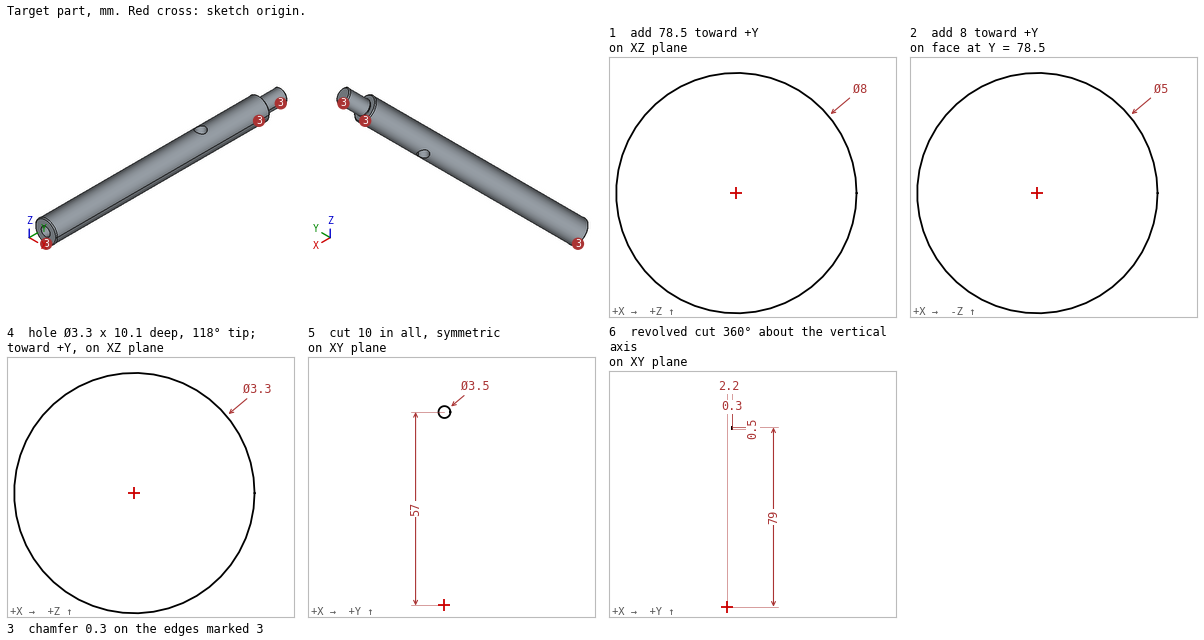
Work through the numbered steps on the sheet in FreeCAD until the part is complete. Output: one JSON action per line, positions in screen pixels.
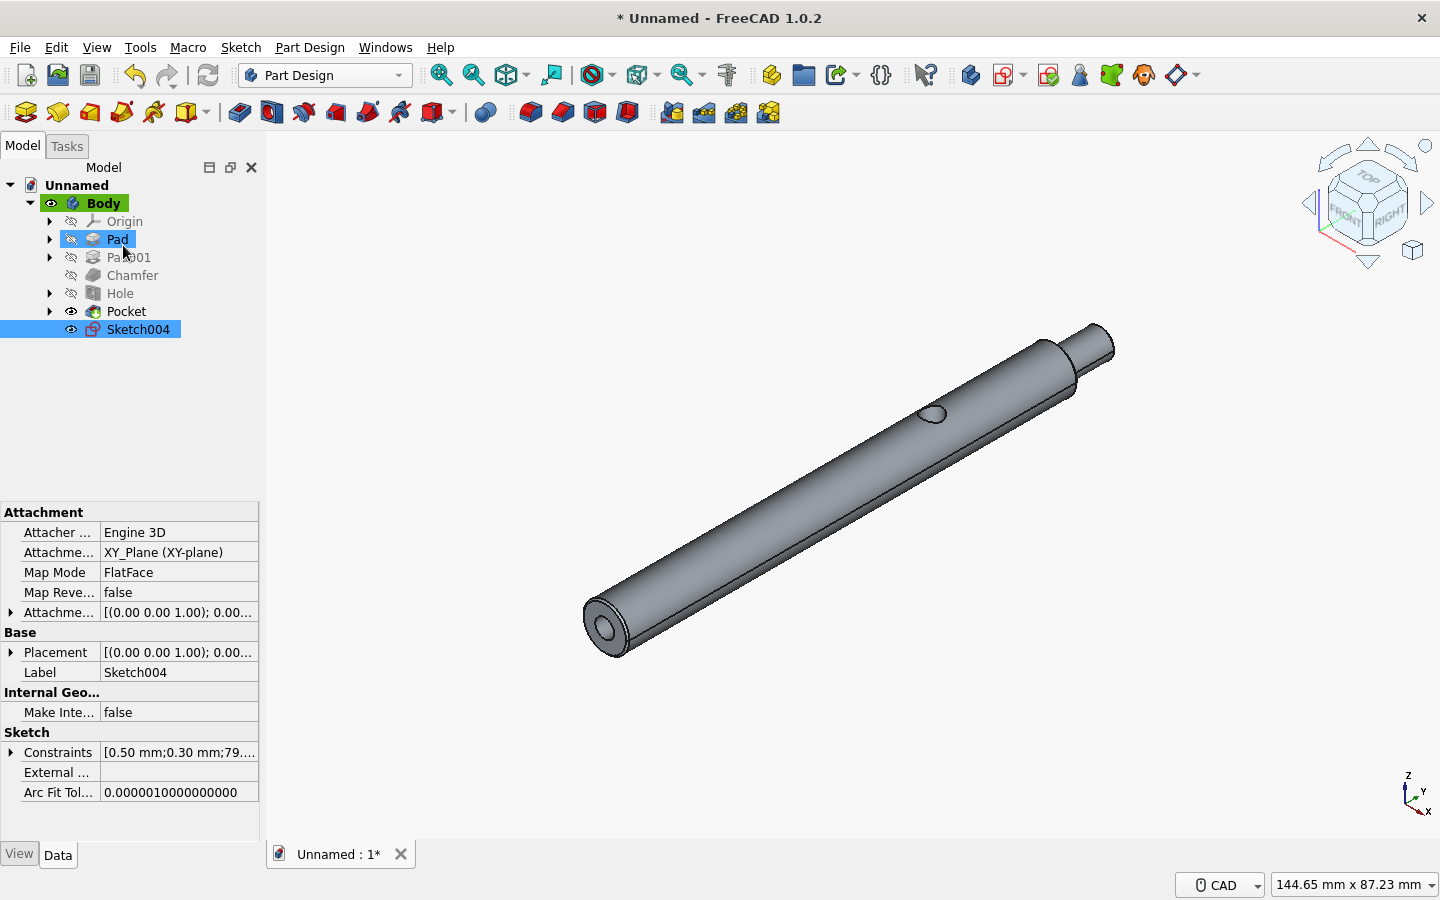
{"action": "left_click", "coordinate": [304, 112]}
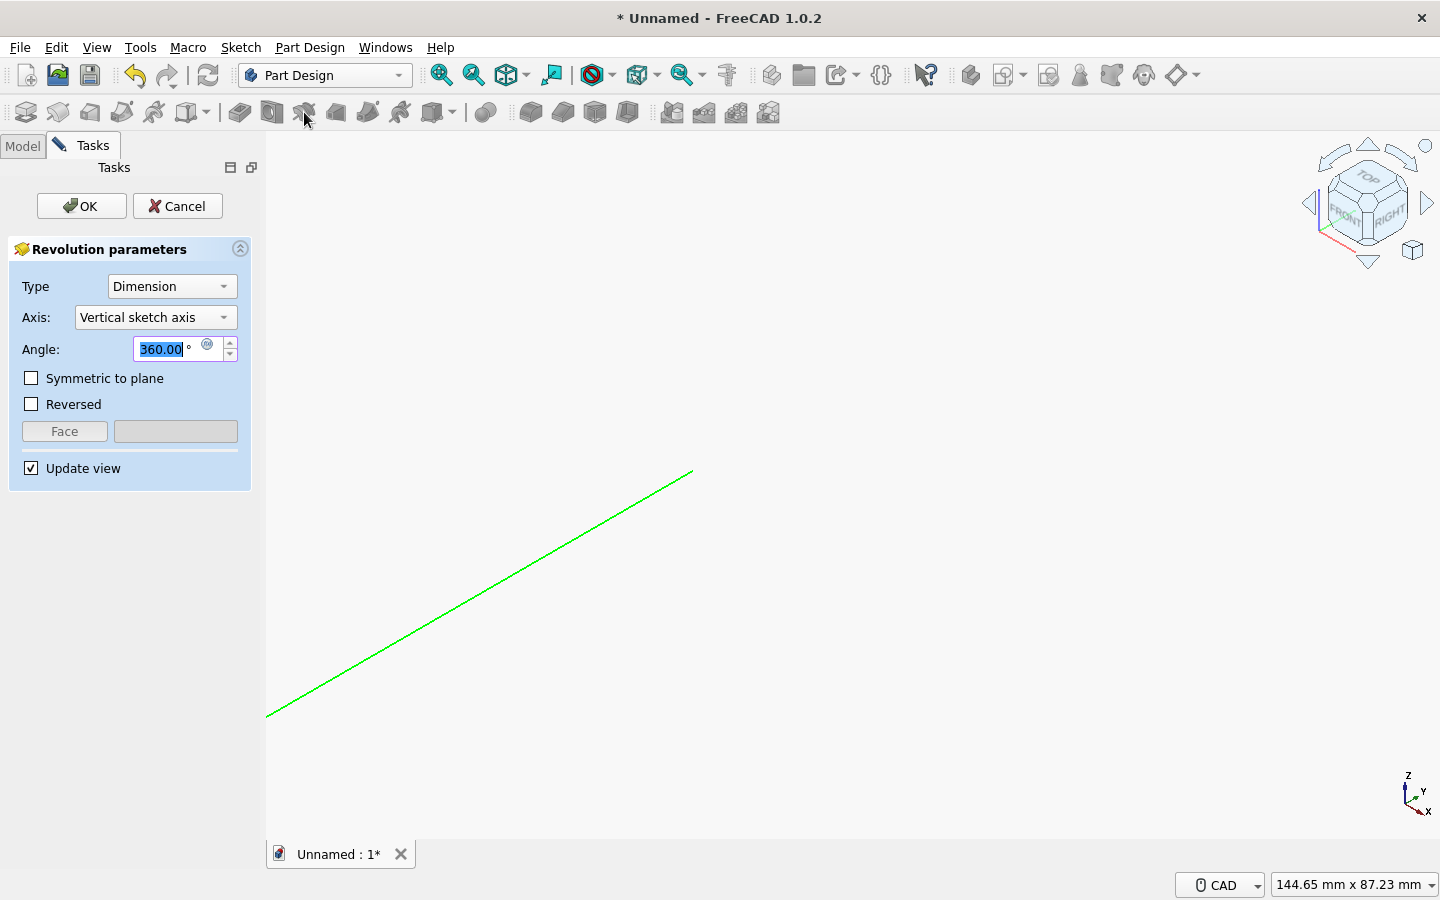
{"action": "left_click", "coordinate": [82, 206]}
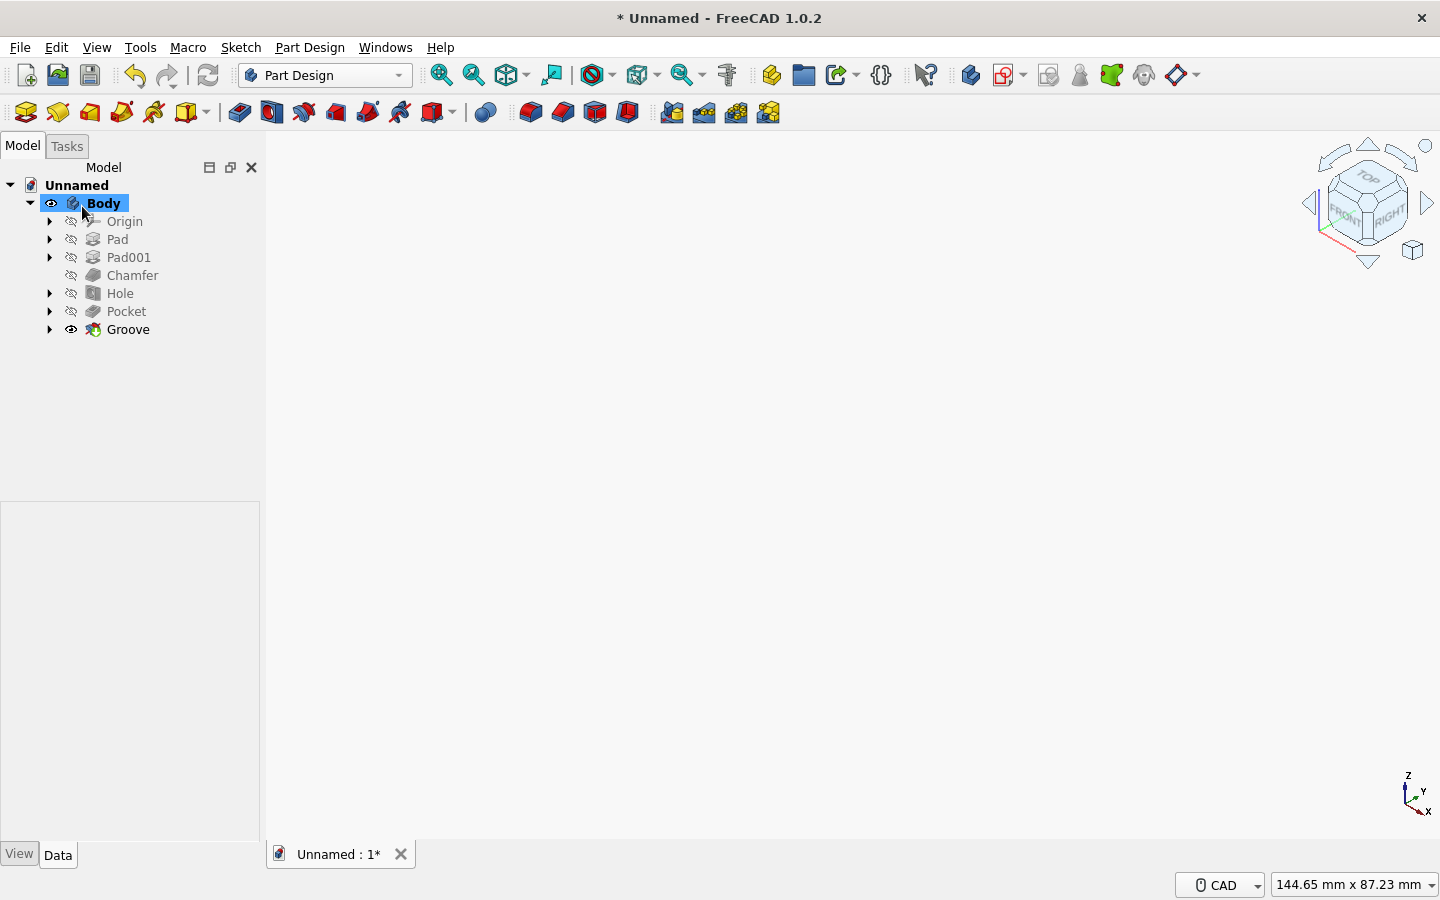
{"action": "key", "text": "v f"}